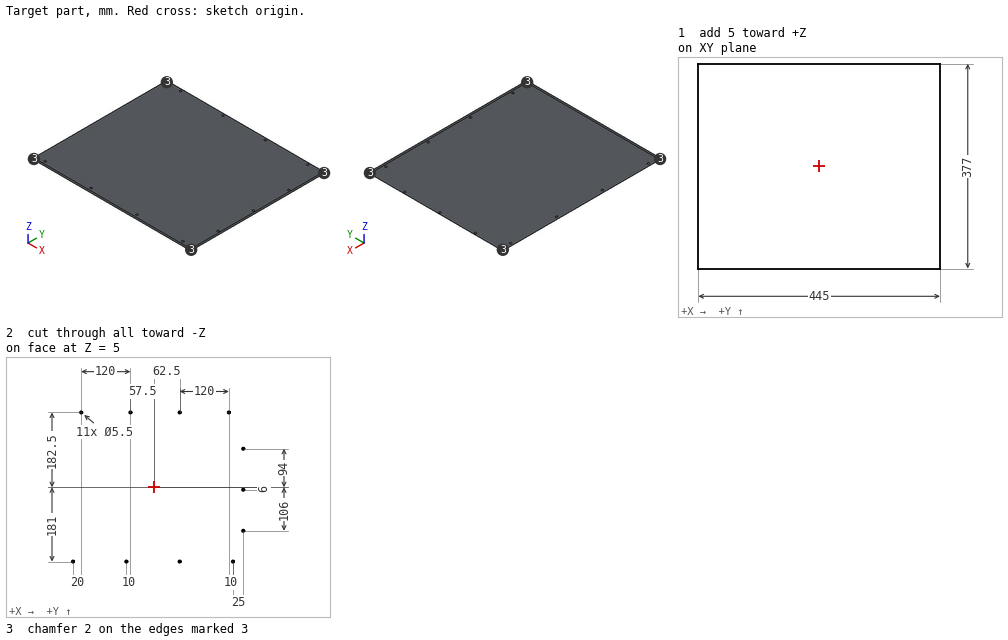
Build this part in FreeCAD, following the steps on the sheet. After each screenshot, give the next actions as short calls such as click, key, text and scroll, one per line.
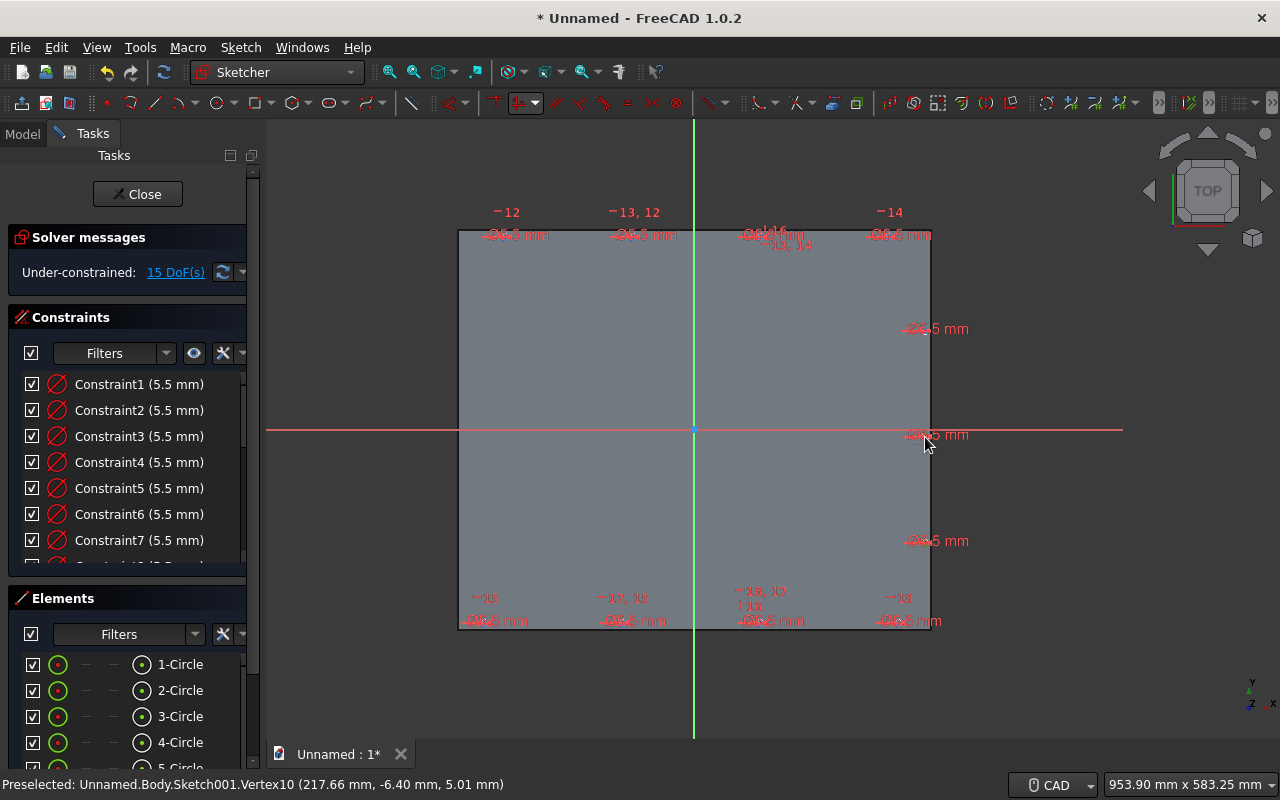
key(v)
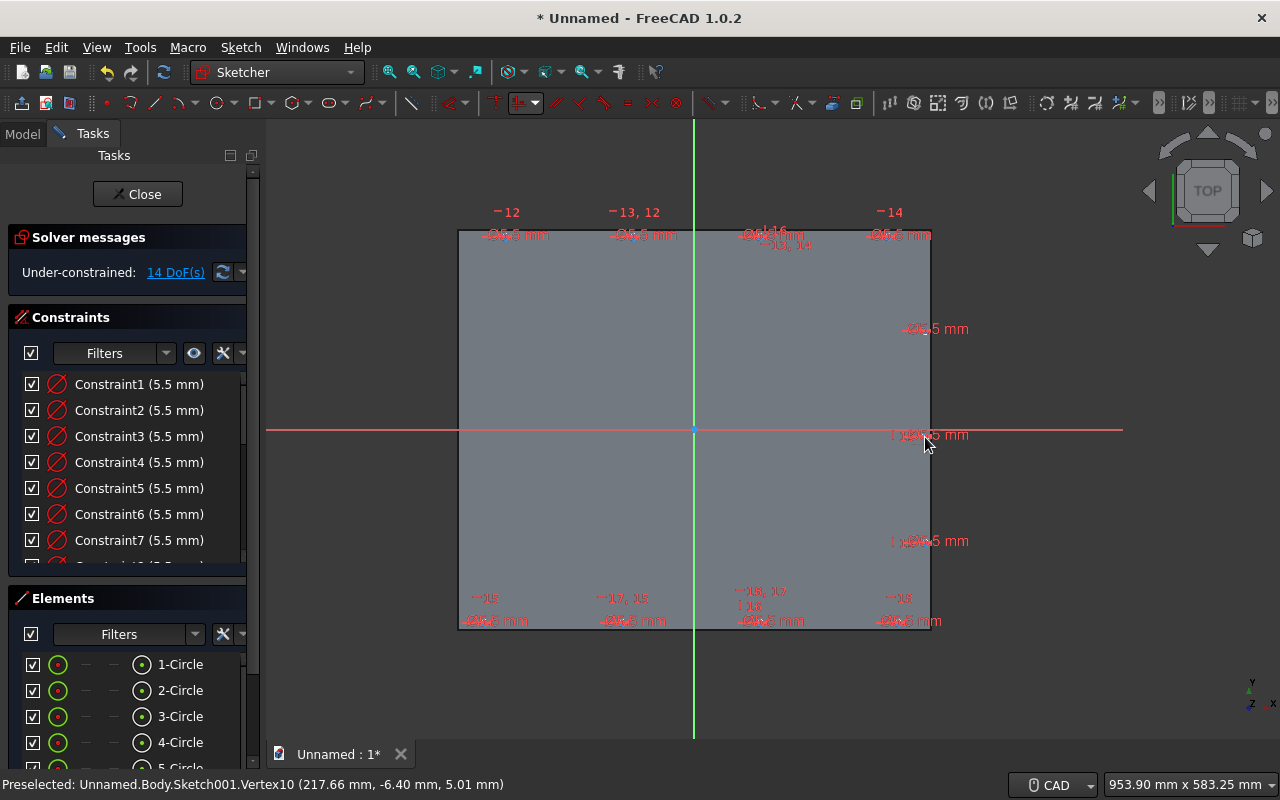
click(925, 437)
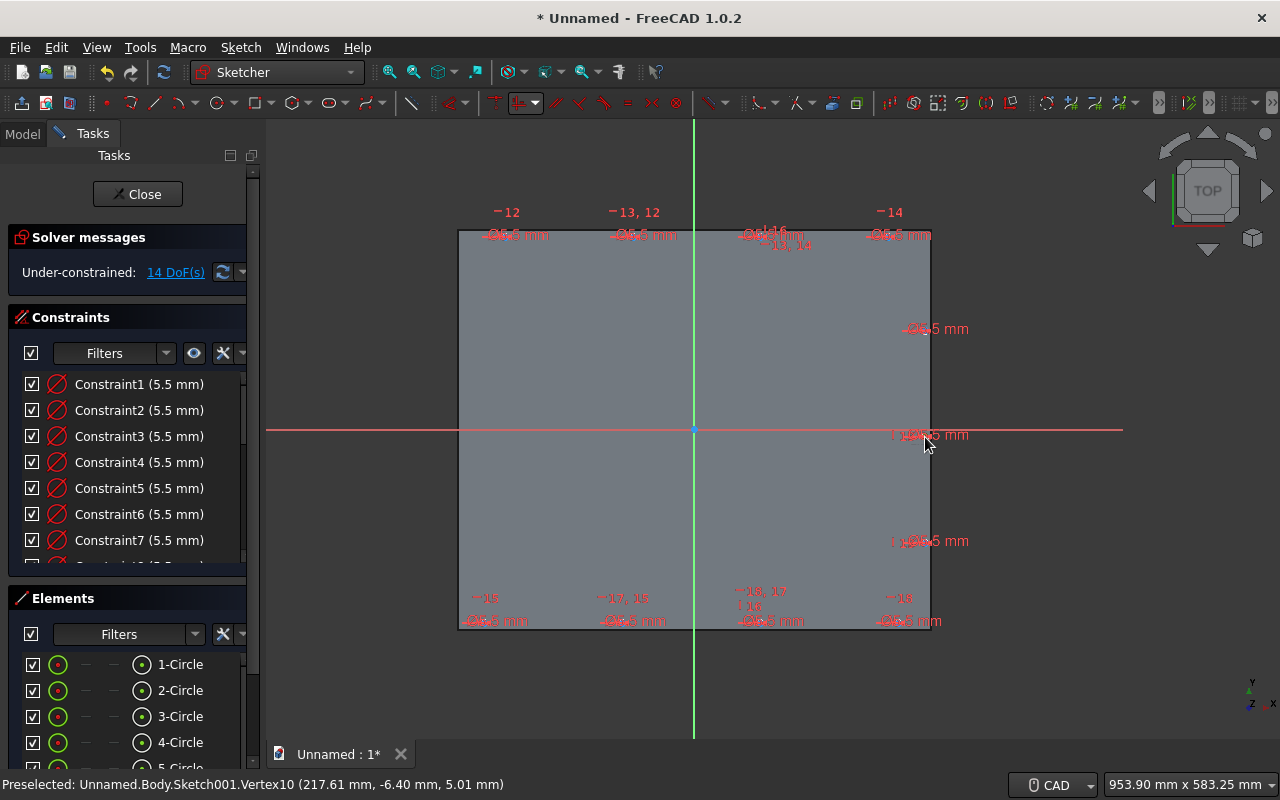
click(925, 331)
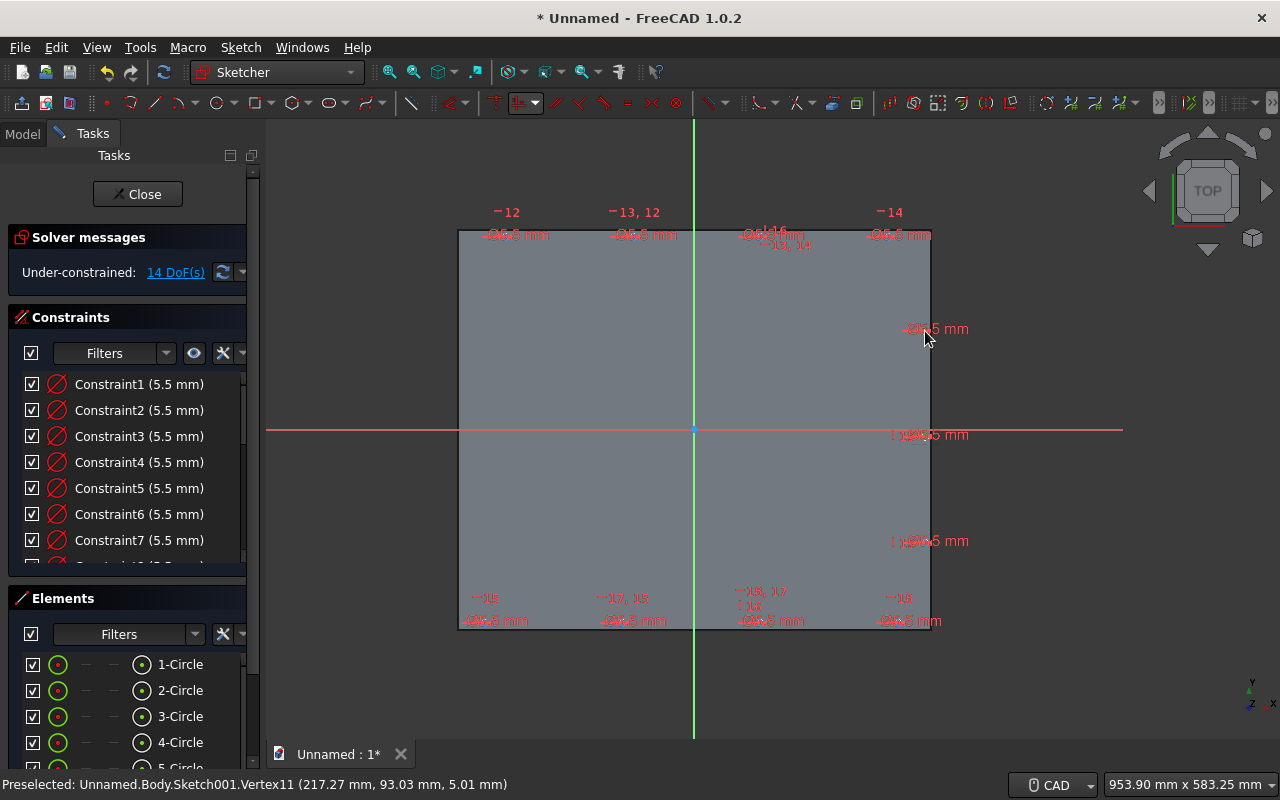
click(538, 104)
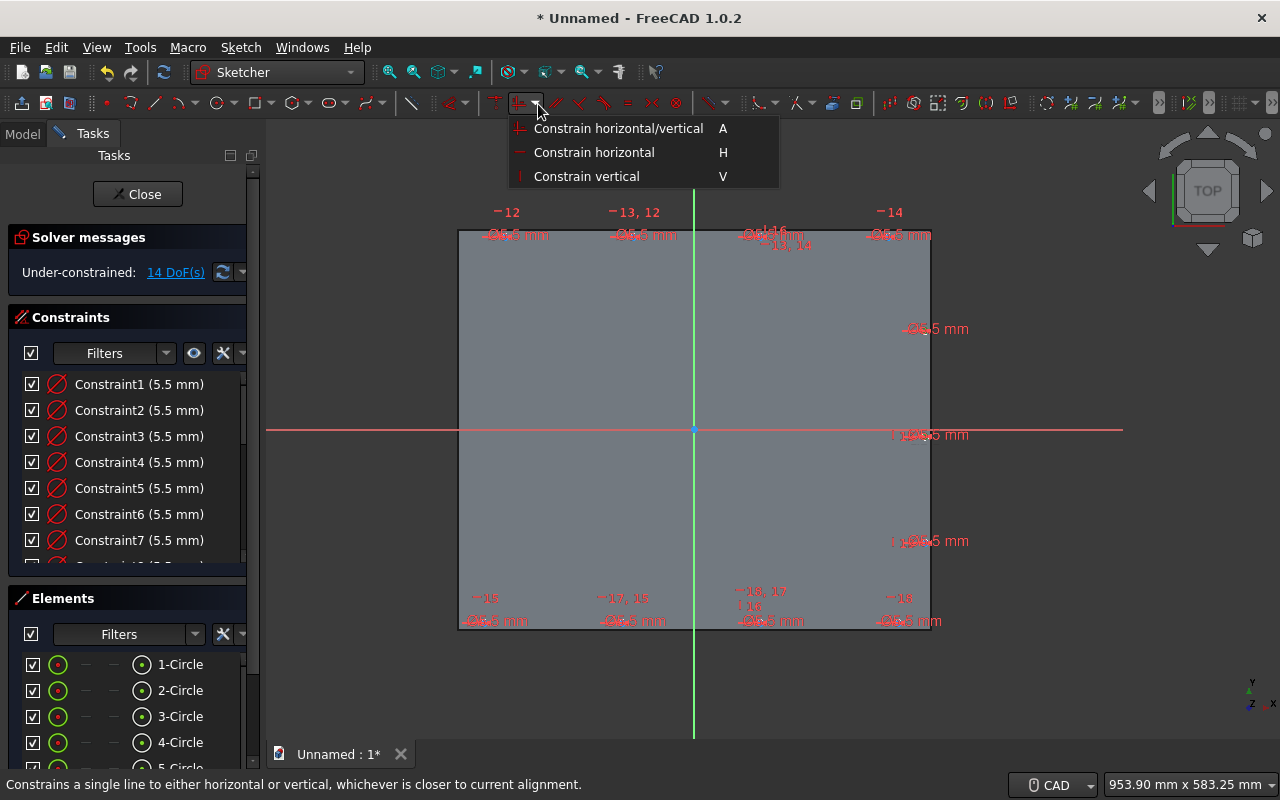
click(644, 176)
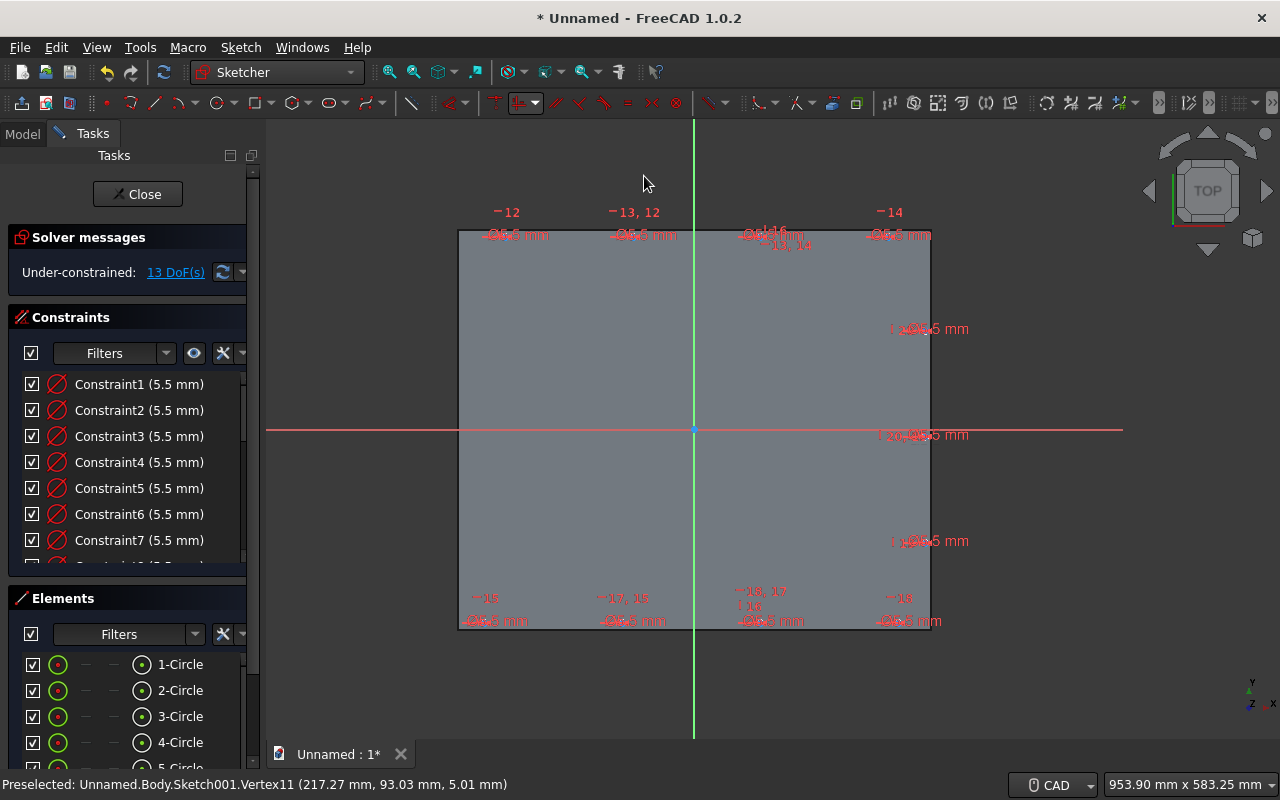
click(450, 104)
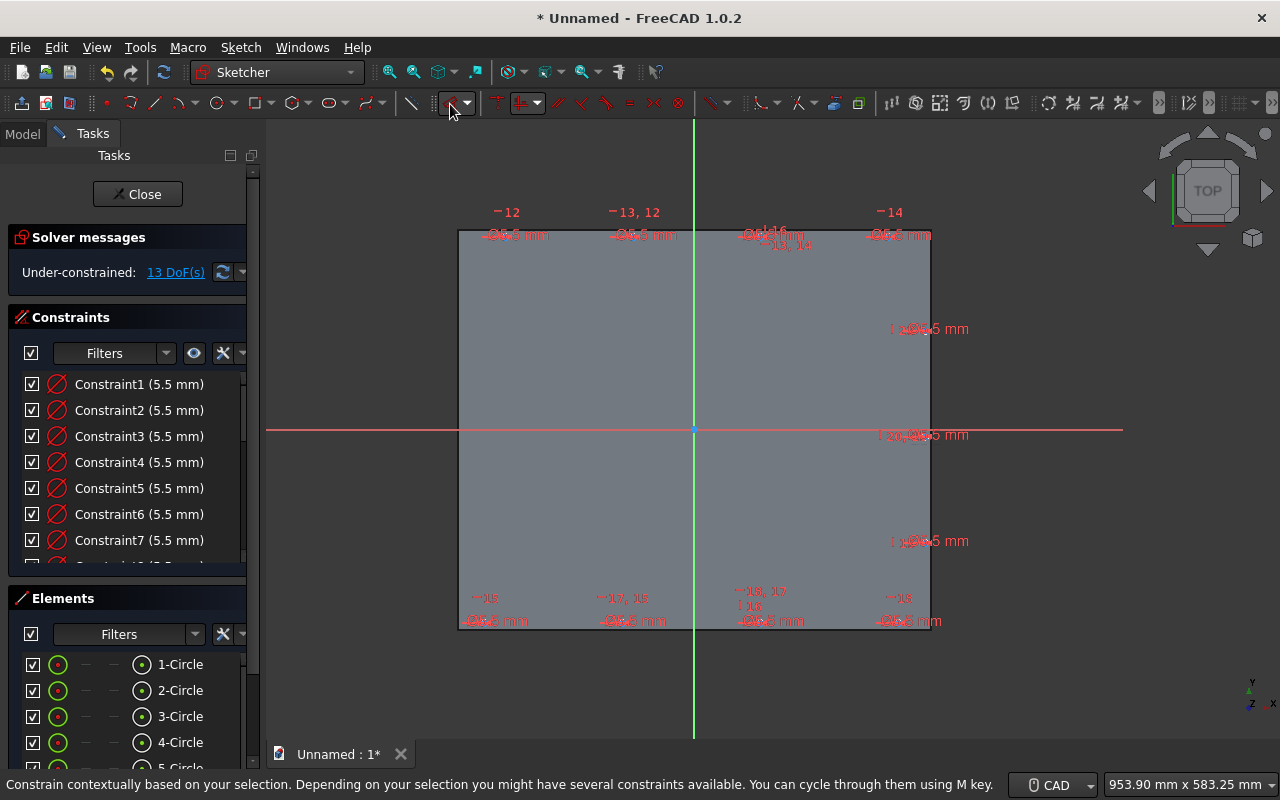
scroll(925, 437, up, 10)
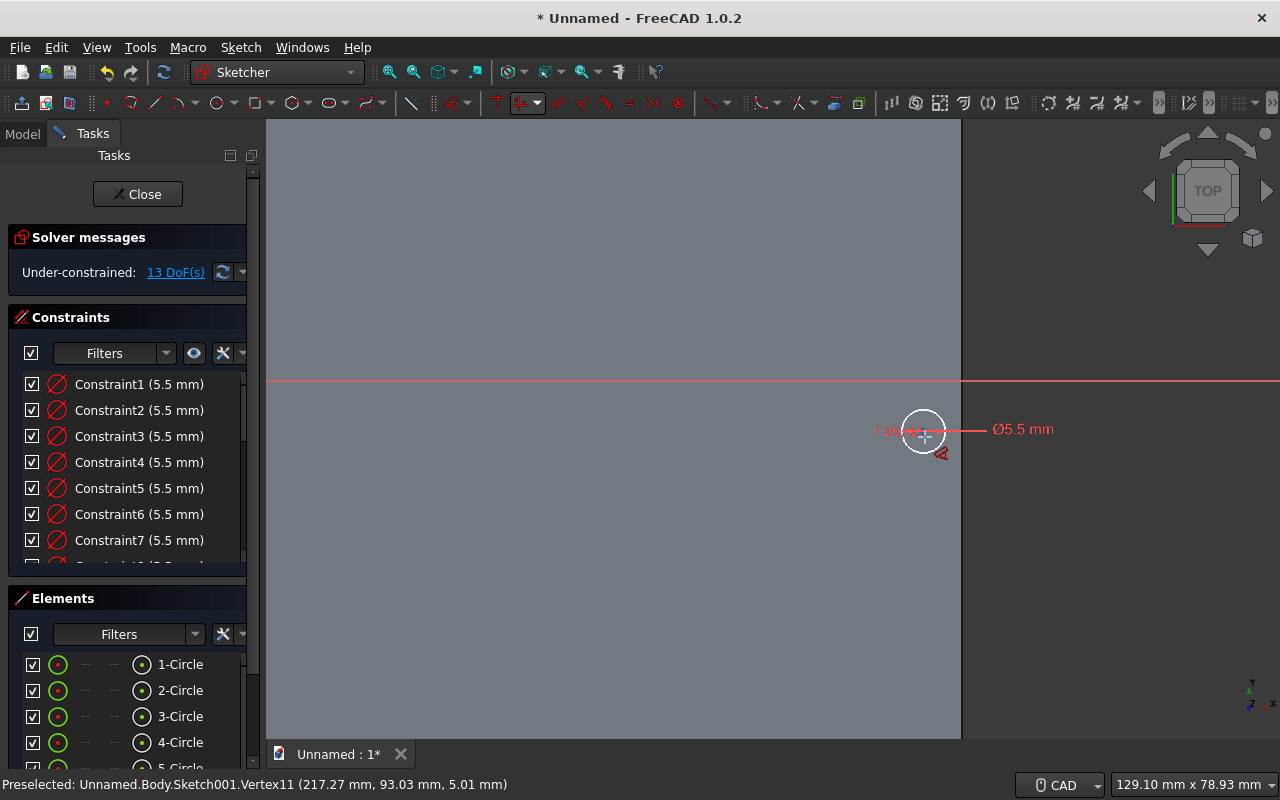
click(924, 431)
click(958, 406)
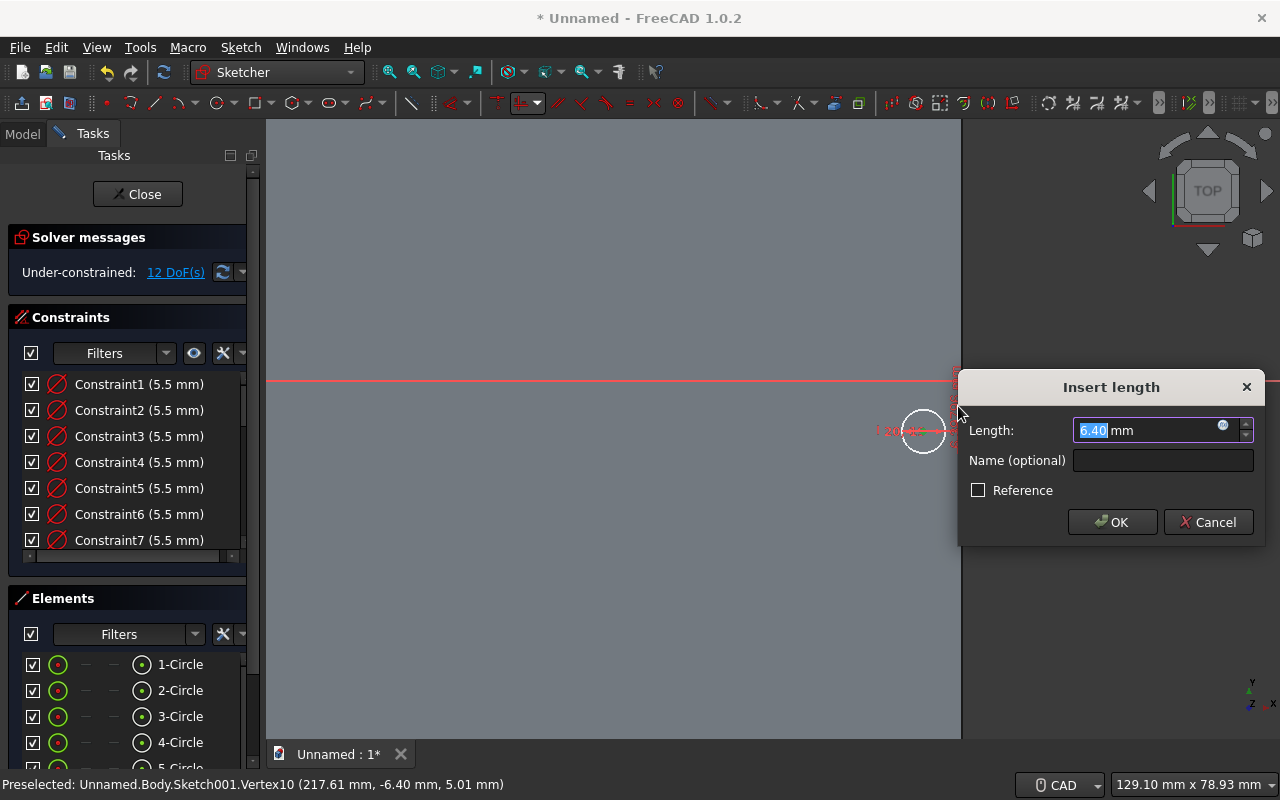
text(6)
key(Return)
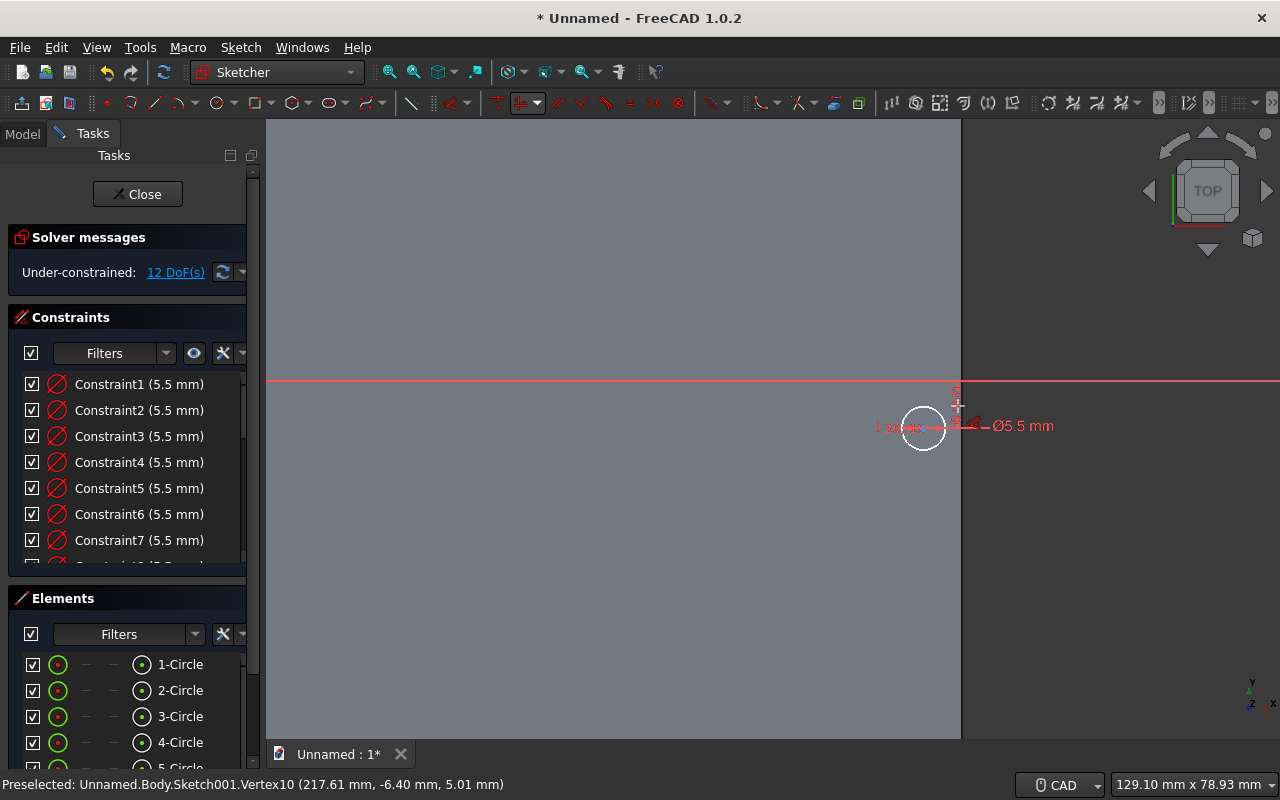
scroll(925, 437, down, 10)